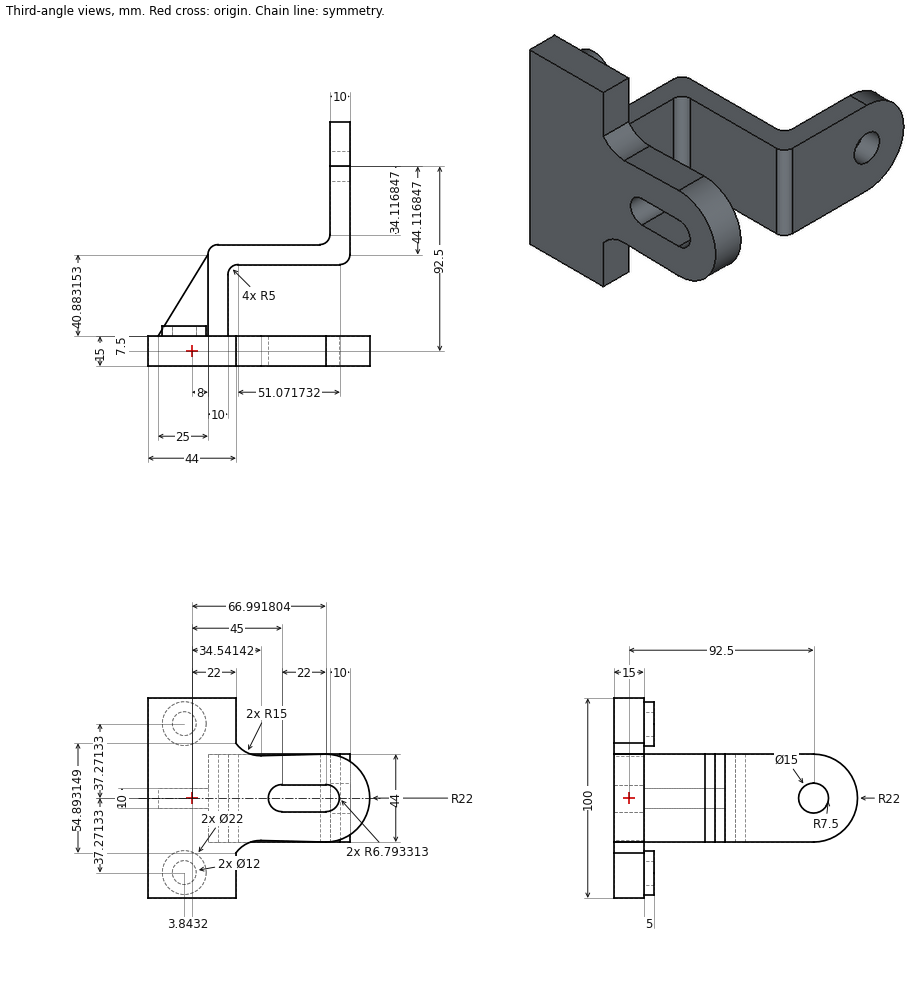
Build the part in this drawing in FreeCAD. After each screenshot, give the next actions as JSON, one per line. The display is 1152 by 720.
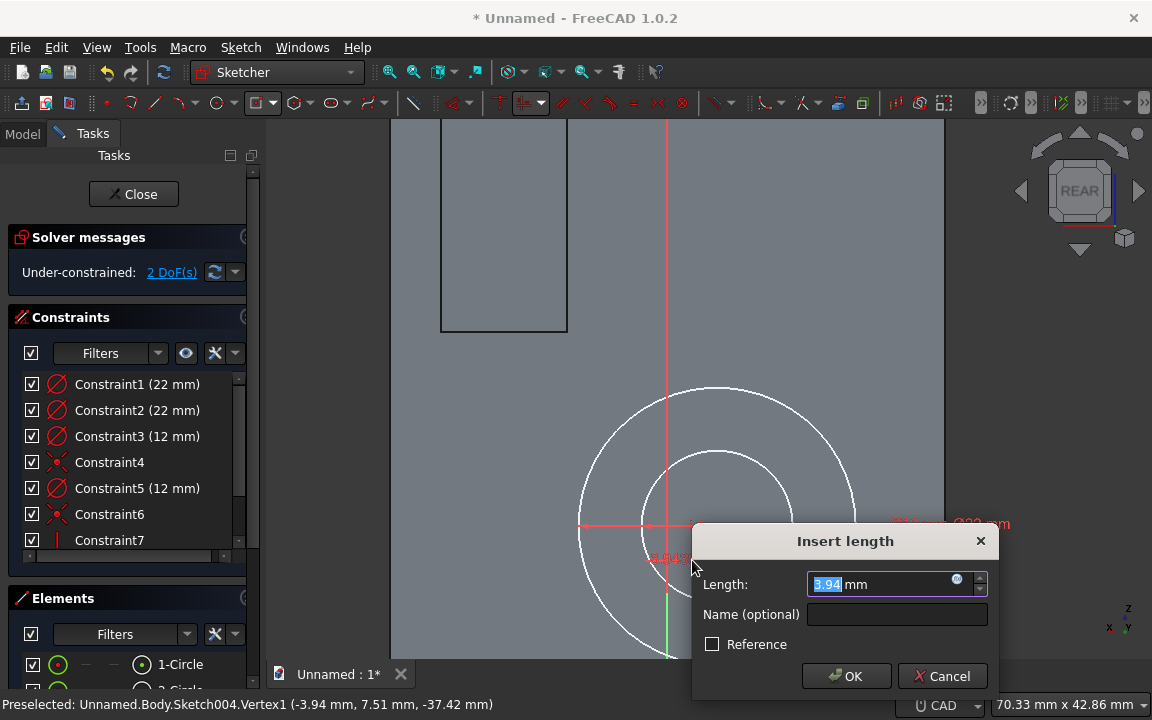
{"action": "type", "text": "3.8432"}
{"action": "key", "text": "Return"}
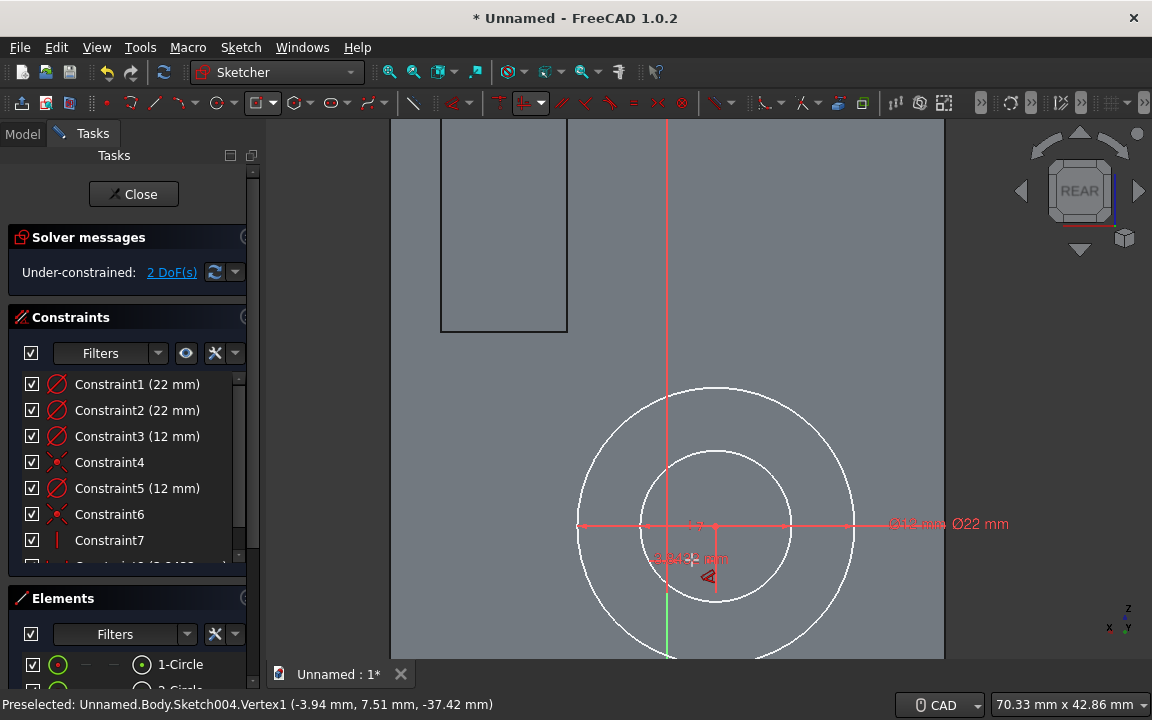
{"action": "scroll", "coordinate": [608, 533], "scroll_direction": "down", "scroll_amount": 6}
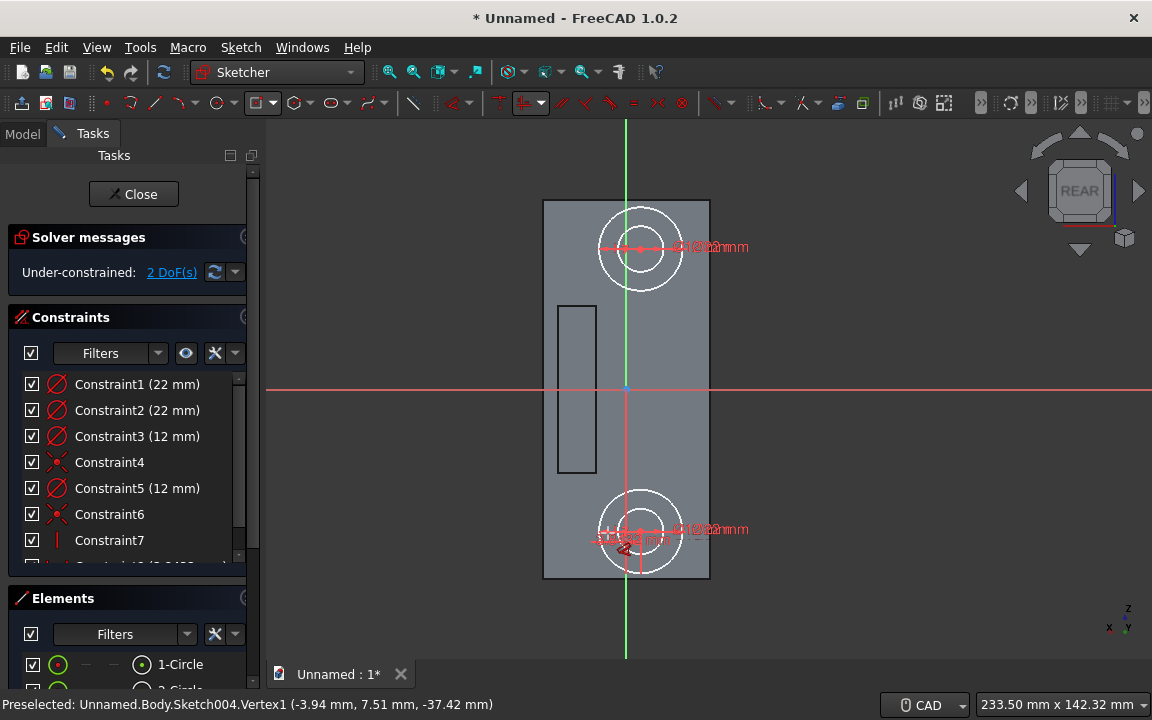
{"action": "left_click", "coordinate": [641, 532]}
{"action": "left_click", "coordinate": [592, 461]}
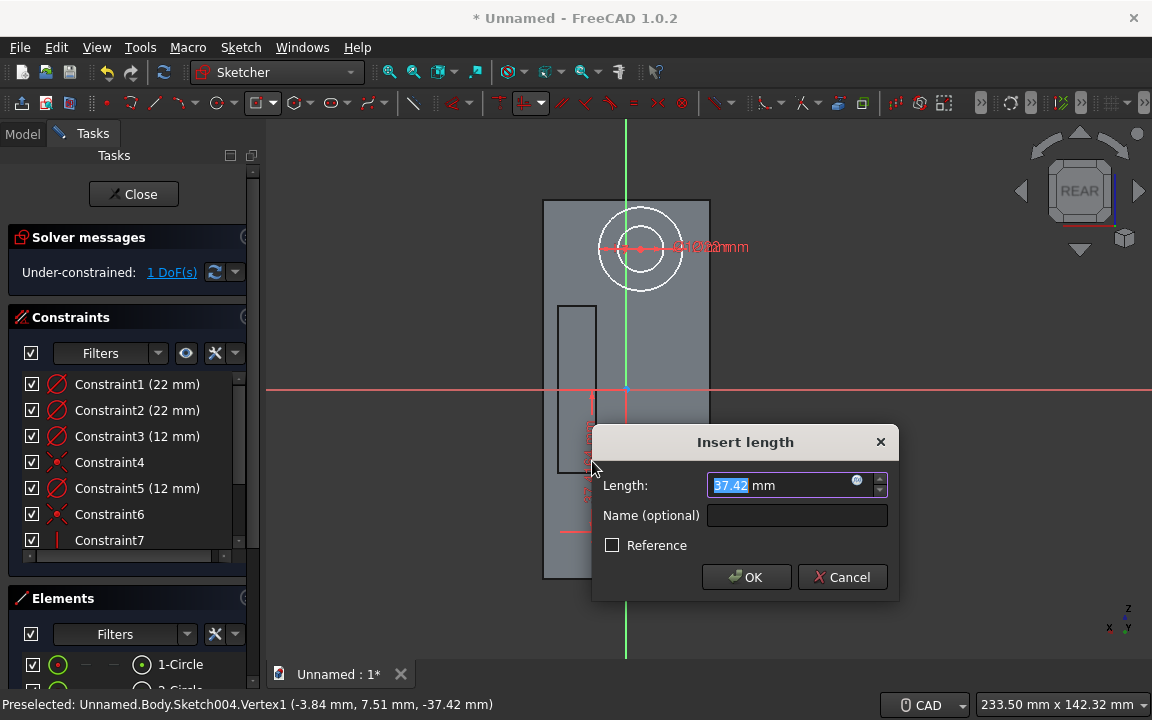
{"action": "type", "text": "37.27133"}
{"action": "key", "text": "Return"}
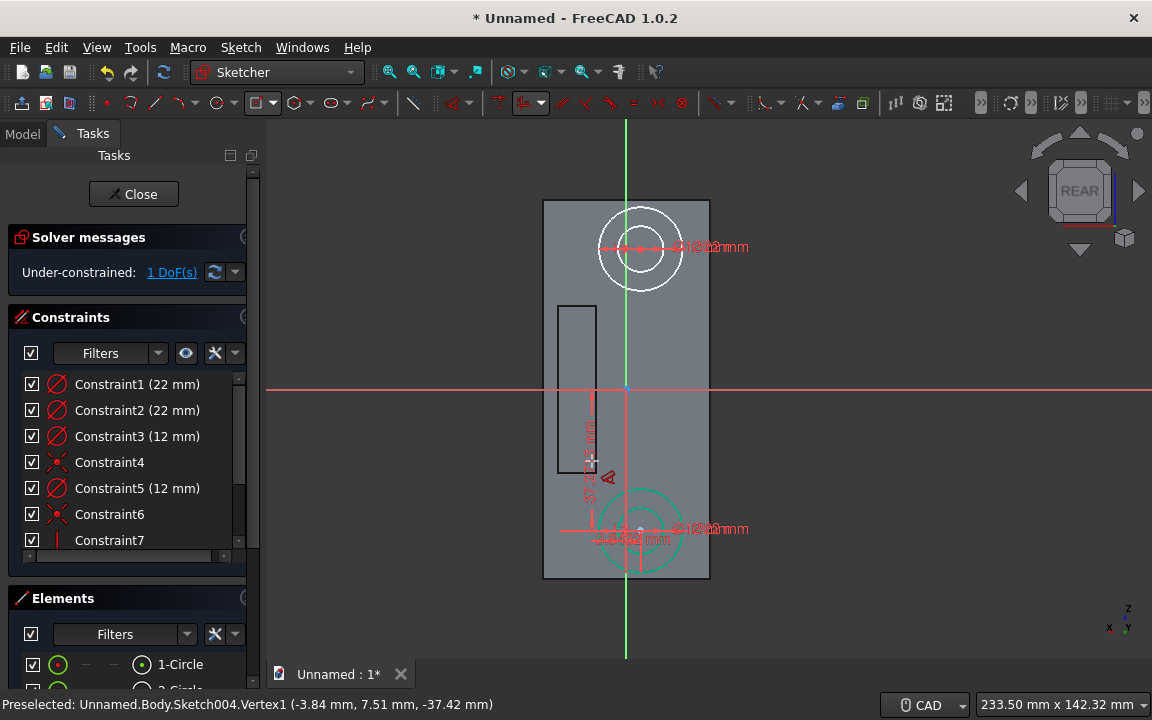
{"action": "left_click", "coordinate": [641, 249]}
{"action": "left_click", "coordinate": [592, 319]}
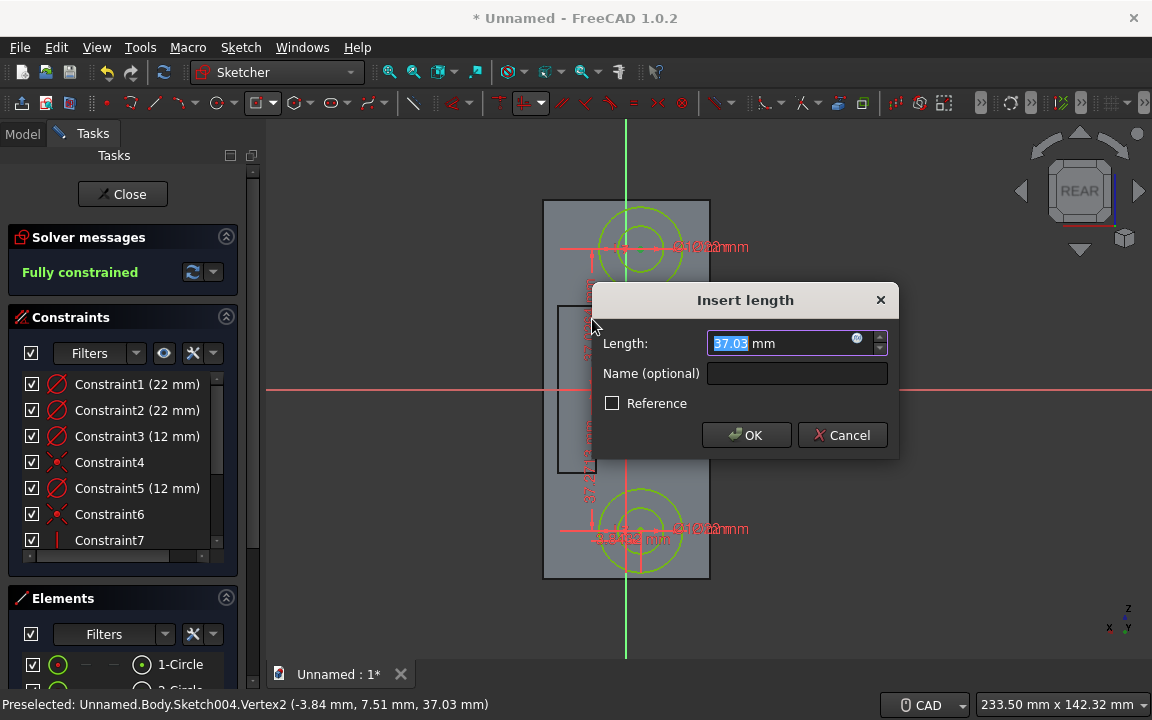
{"action": "type", "text": "37.27133"}
{"action": "key", "text": "Return"}
{"action": "key", "text": "Escape"}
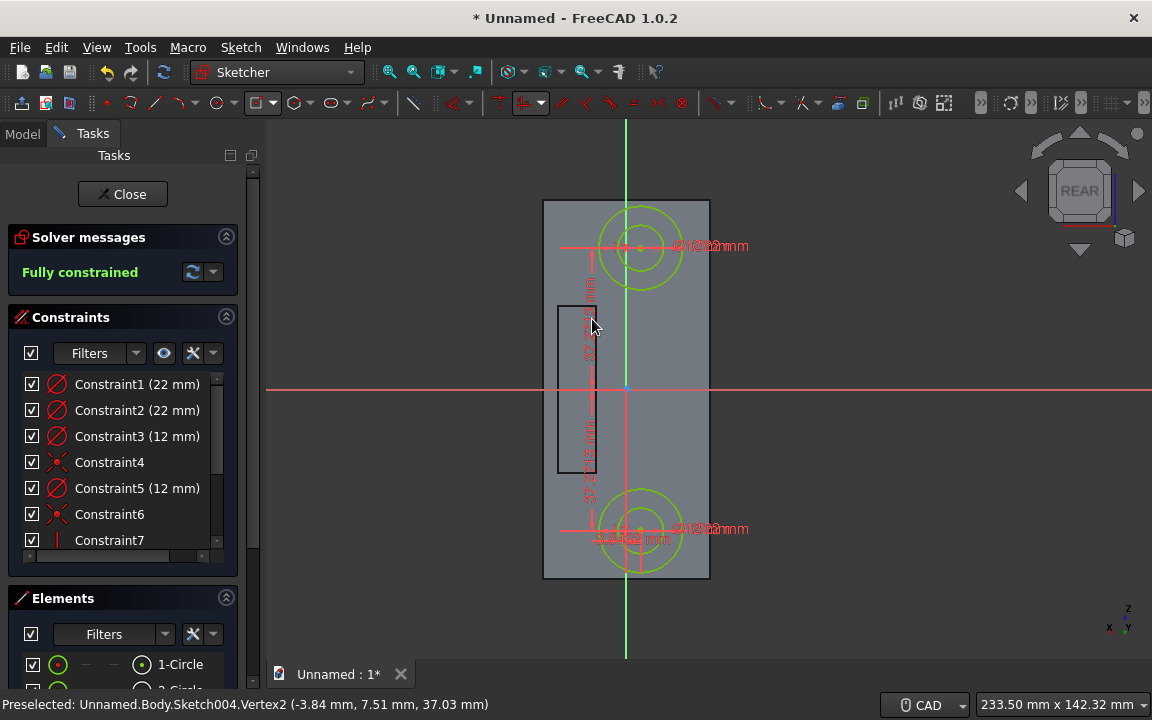
{"action": "left_click", "coordinate": [123, 194]}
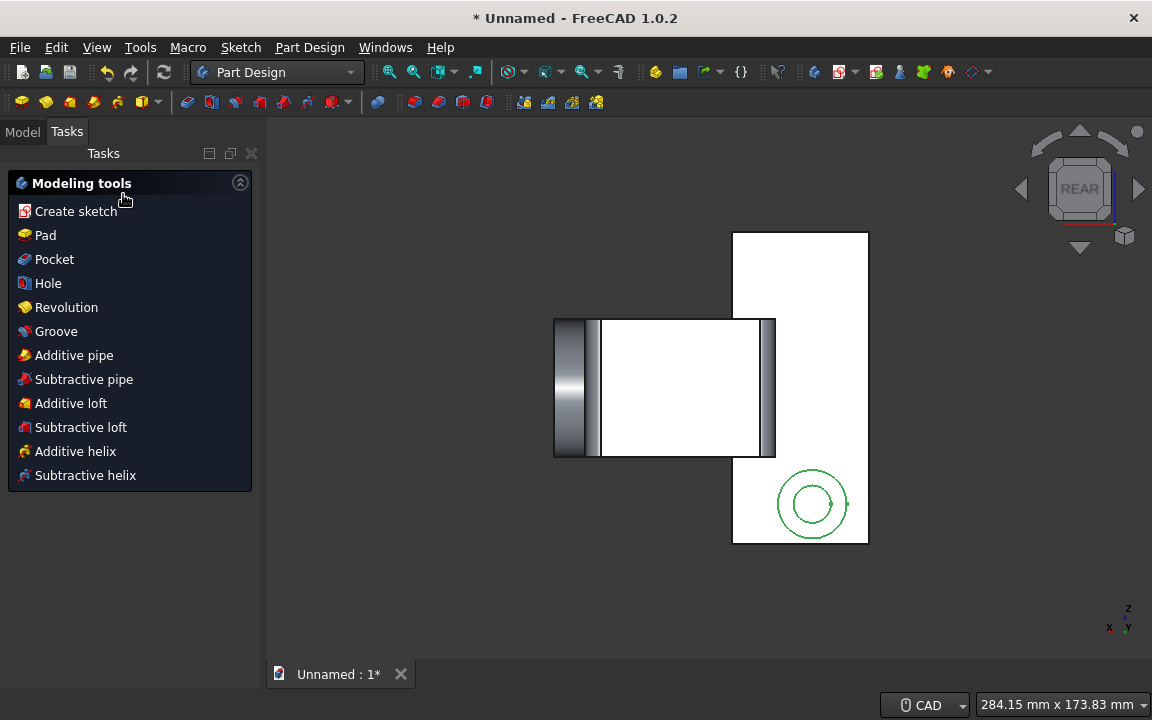
{"action": "left_click", "coordinate": [22, 102]}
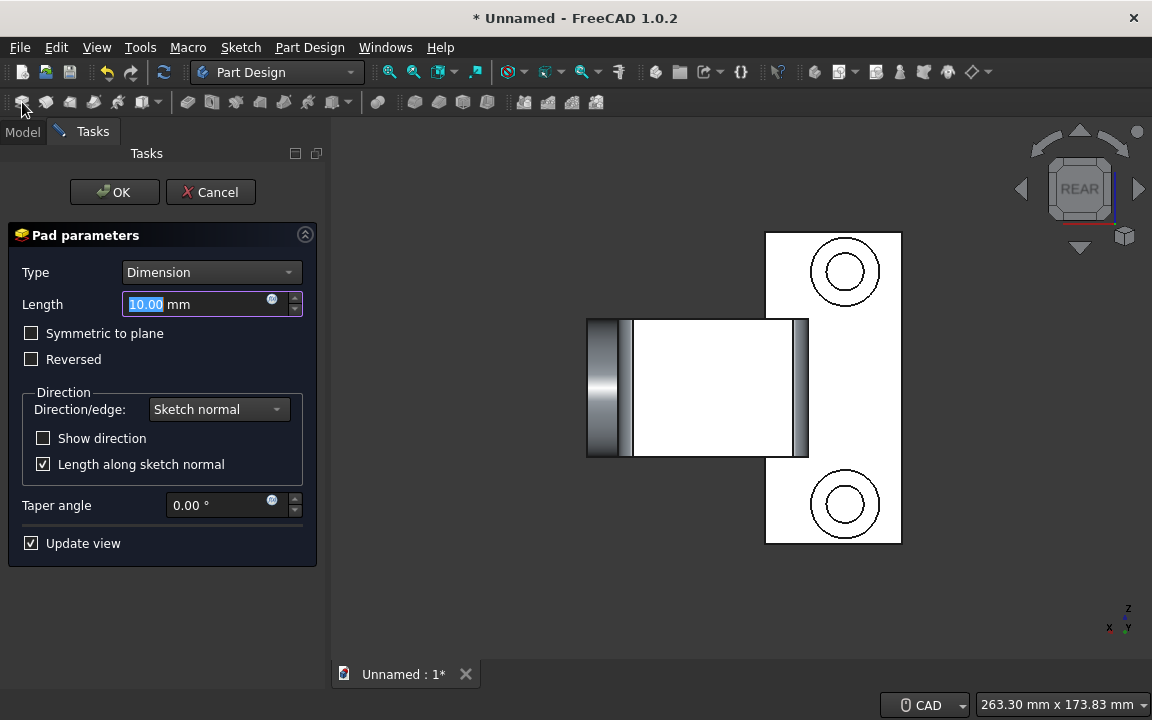
{"action": "type", "text": "5"}
{"action": "key", "text": "Tab"}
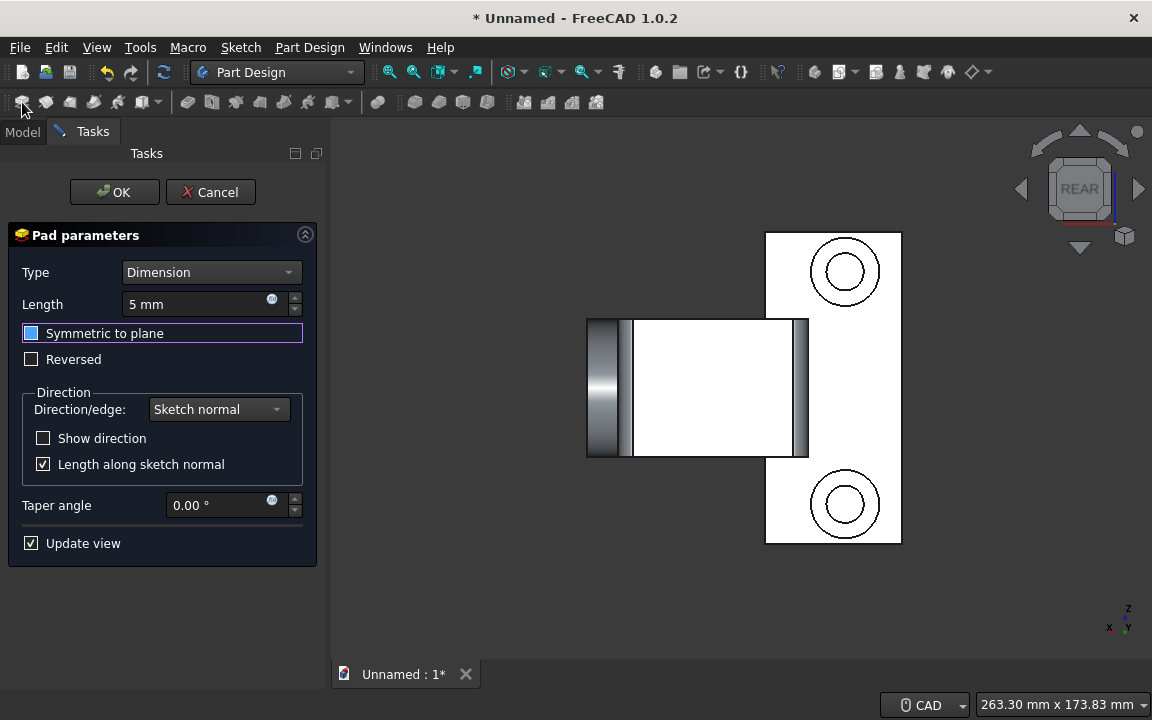
{"action": "left_click", "coordinate": [115, 192]}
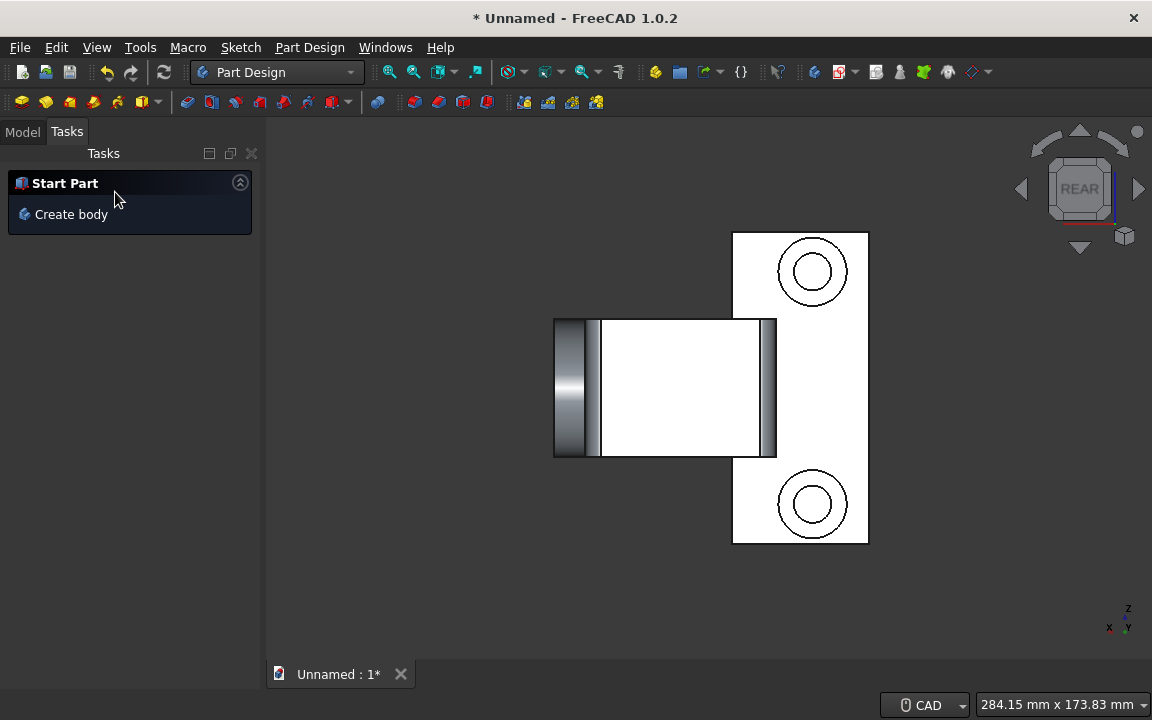
{"action": "left_click", "coordinate": [840, 72]}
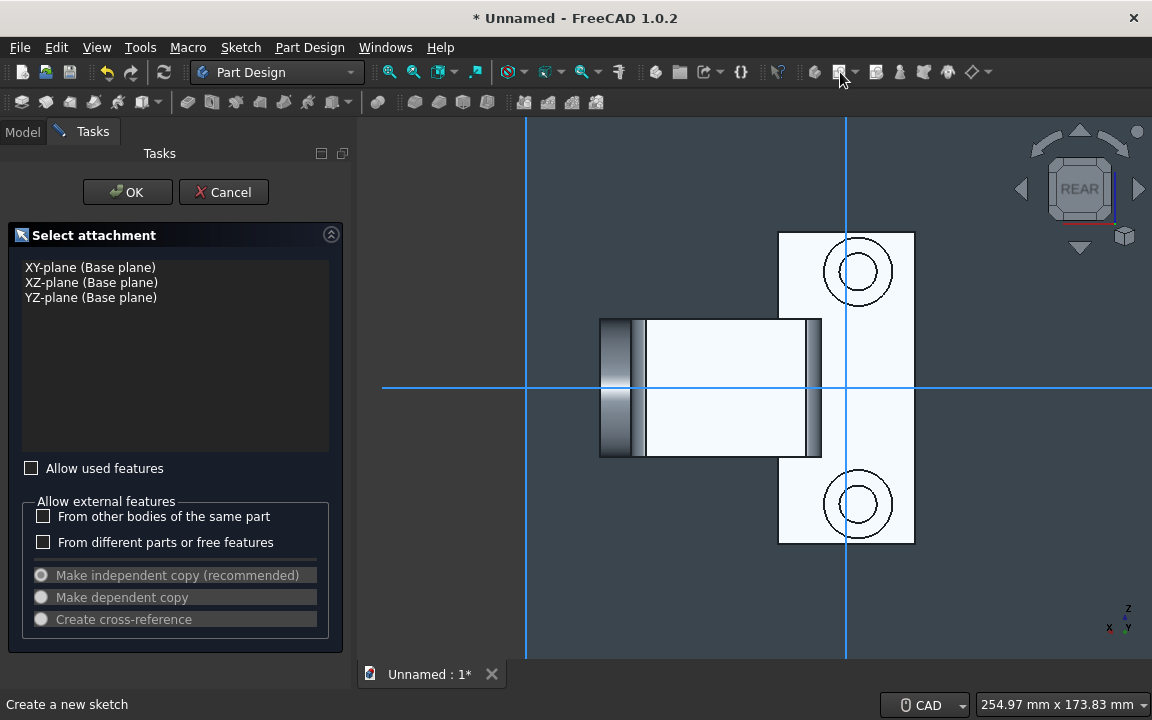
{"action": "left_click", "coordinate": [82, 268]}